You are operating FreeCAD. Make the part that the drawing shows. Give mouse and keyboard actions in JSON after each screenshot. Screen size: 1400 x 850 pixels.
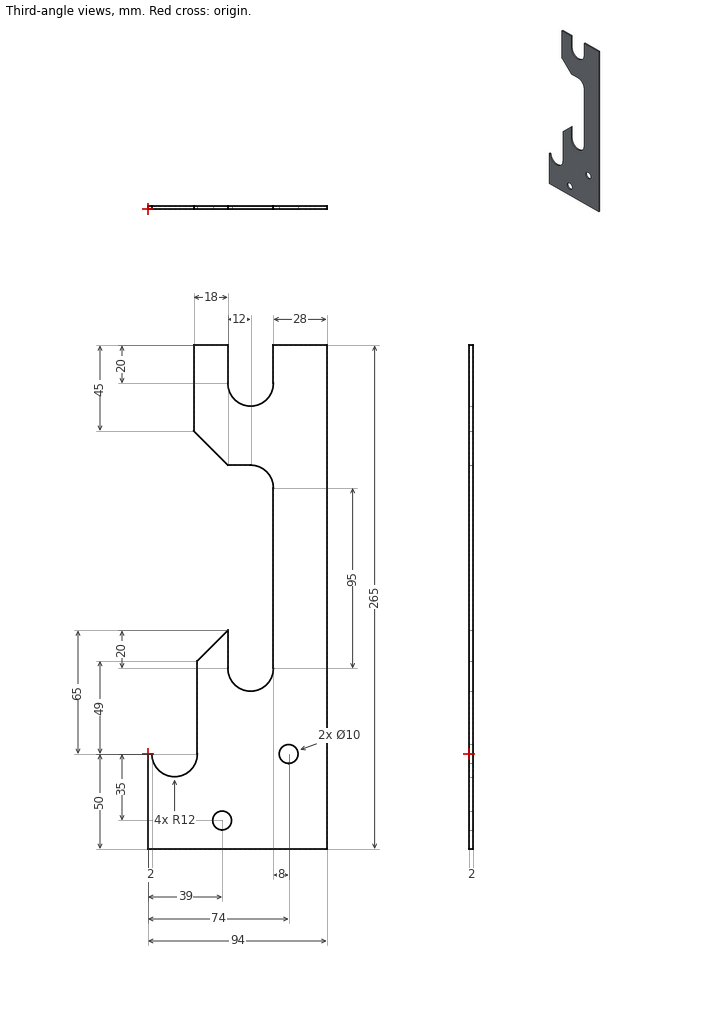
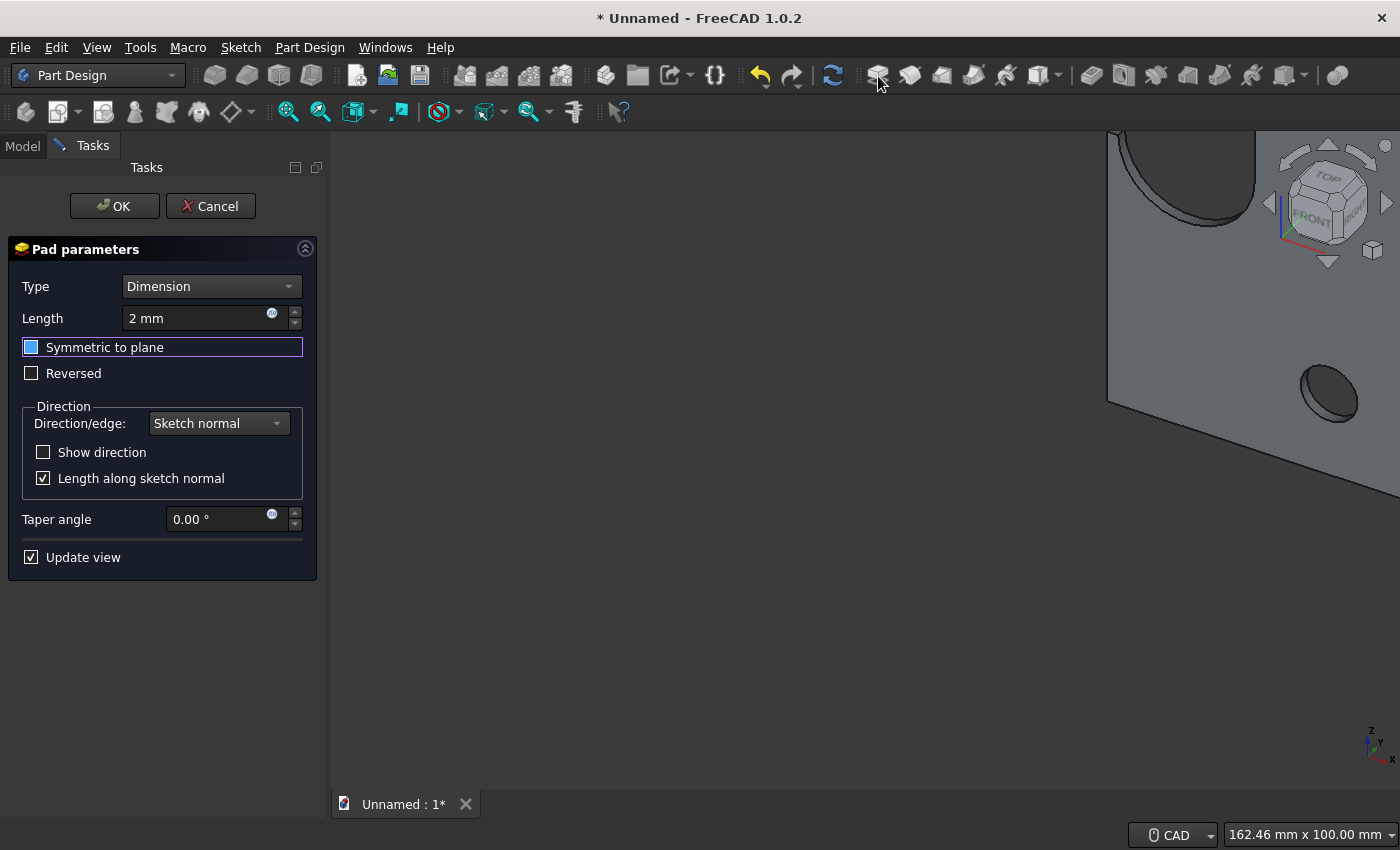
{"action": "left_click", "coordinate": [30, 373]}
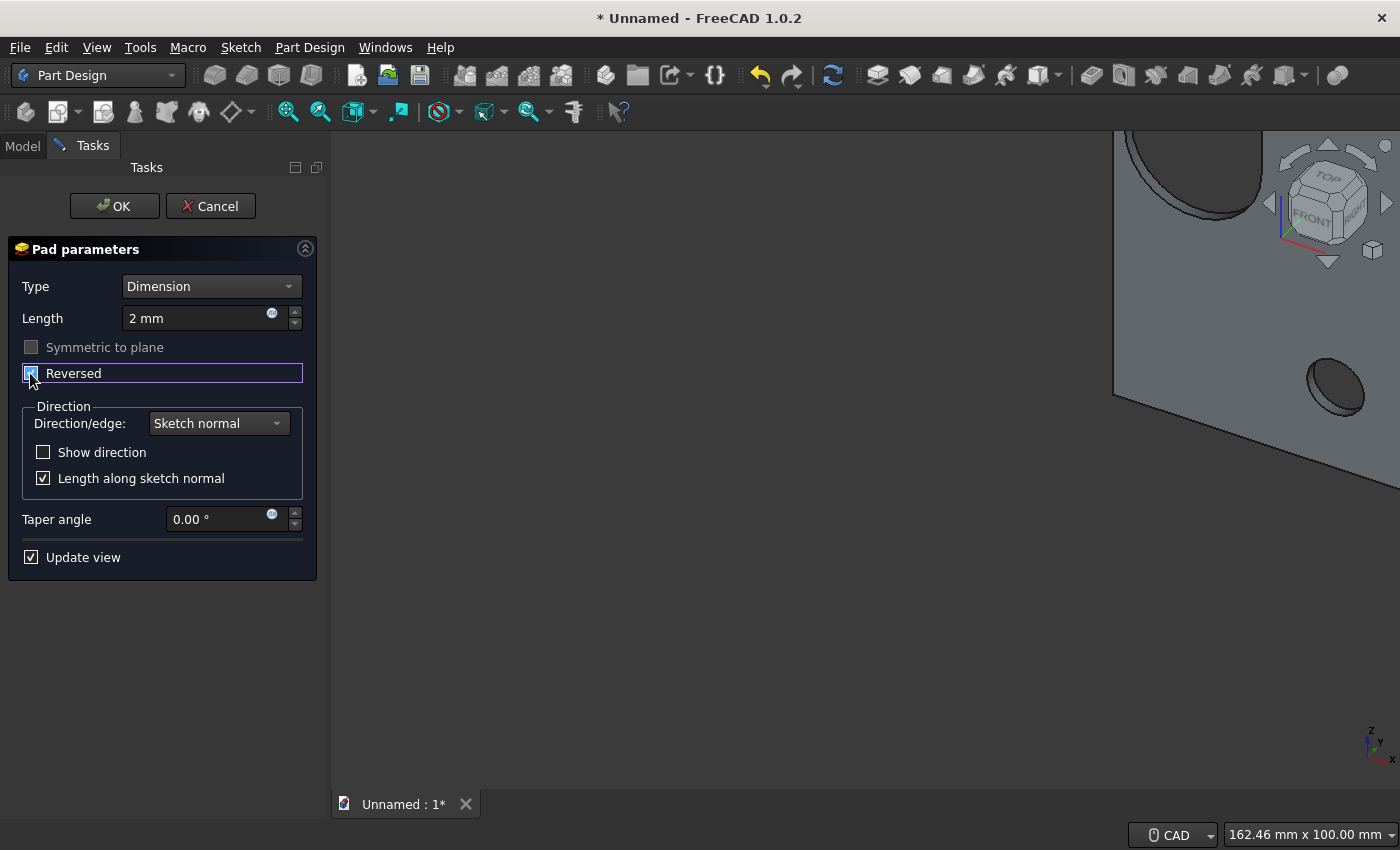
{"action": "left_click", "coordinate": [115, 206]}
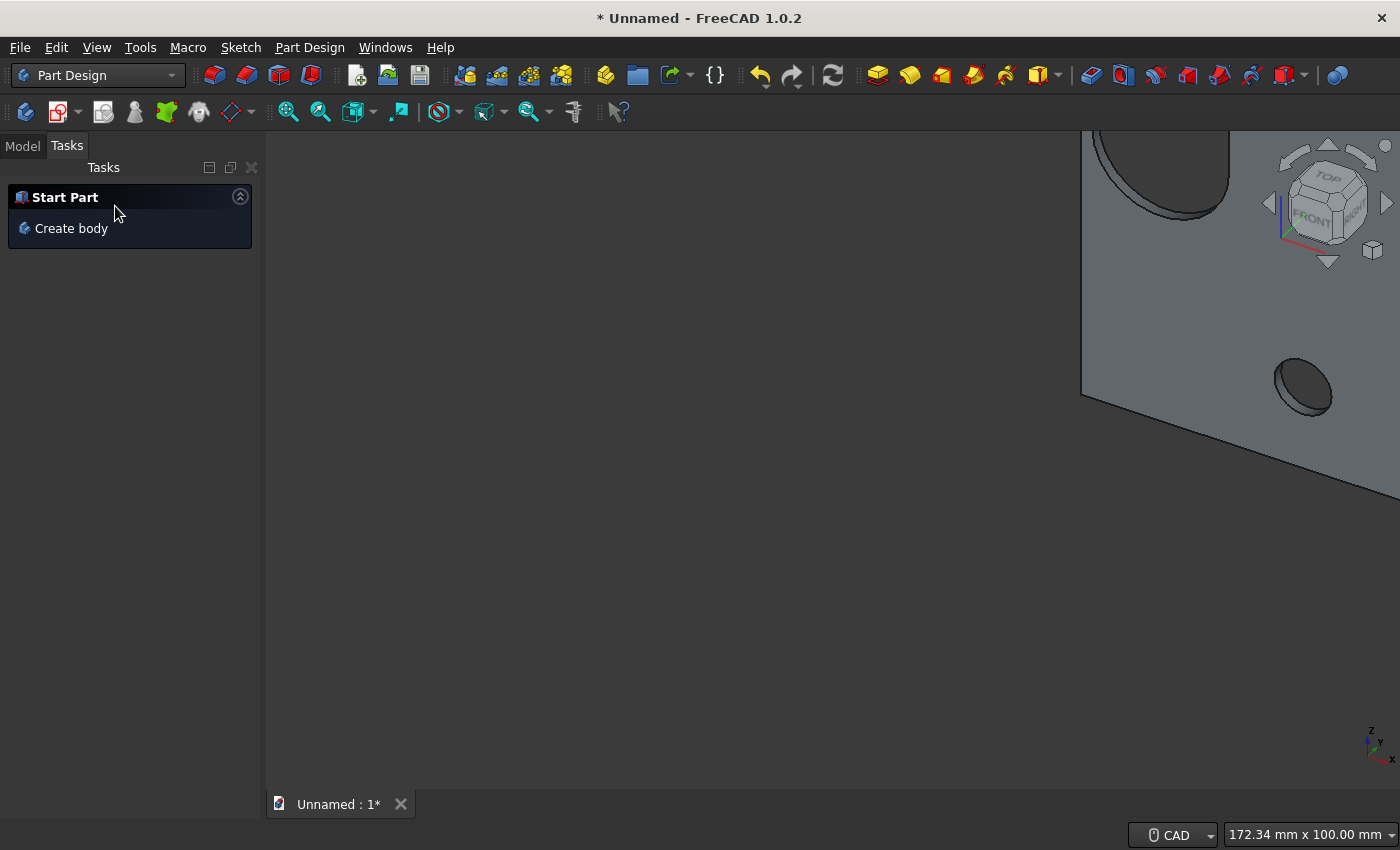
{"action": "key", "text": "0"}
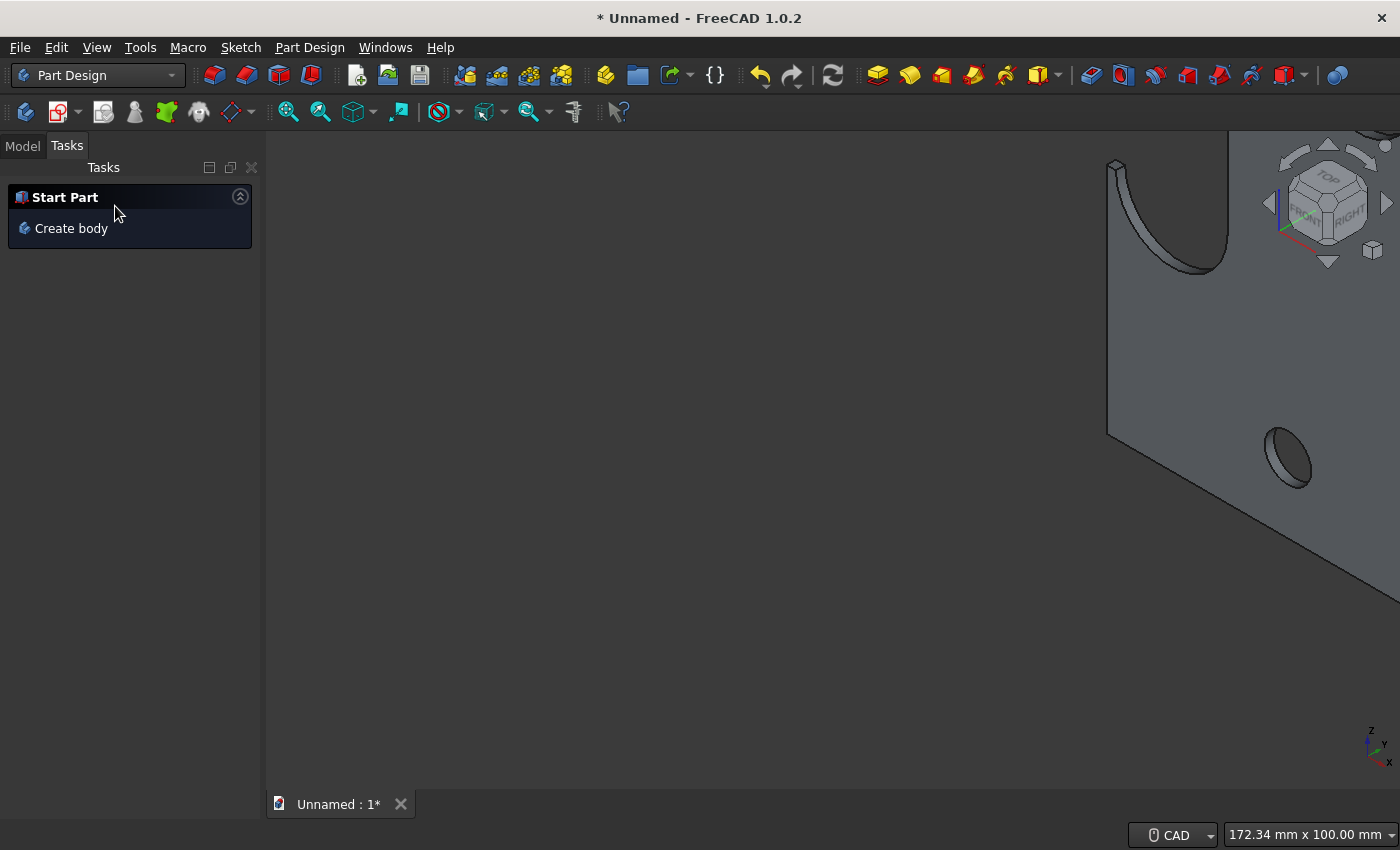
{"action": "key", "text": "v f"}